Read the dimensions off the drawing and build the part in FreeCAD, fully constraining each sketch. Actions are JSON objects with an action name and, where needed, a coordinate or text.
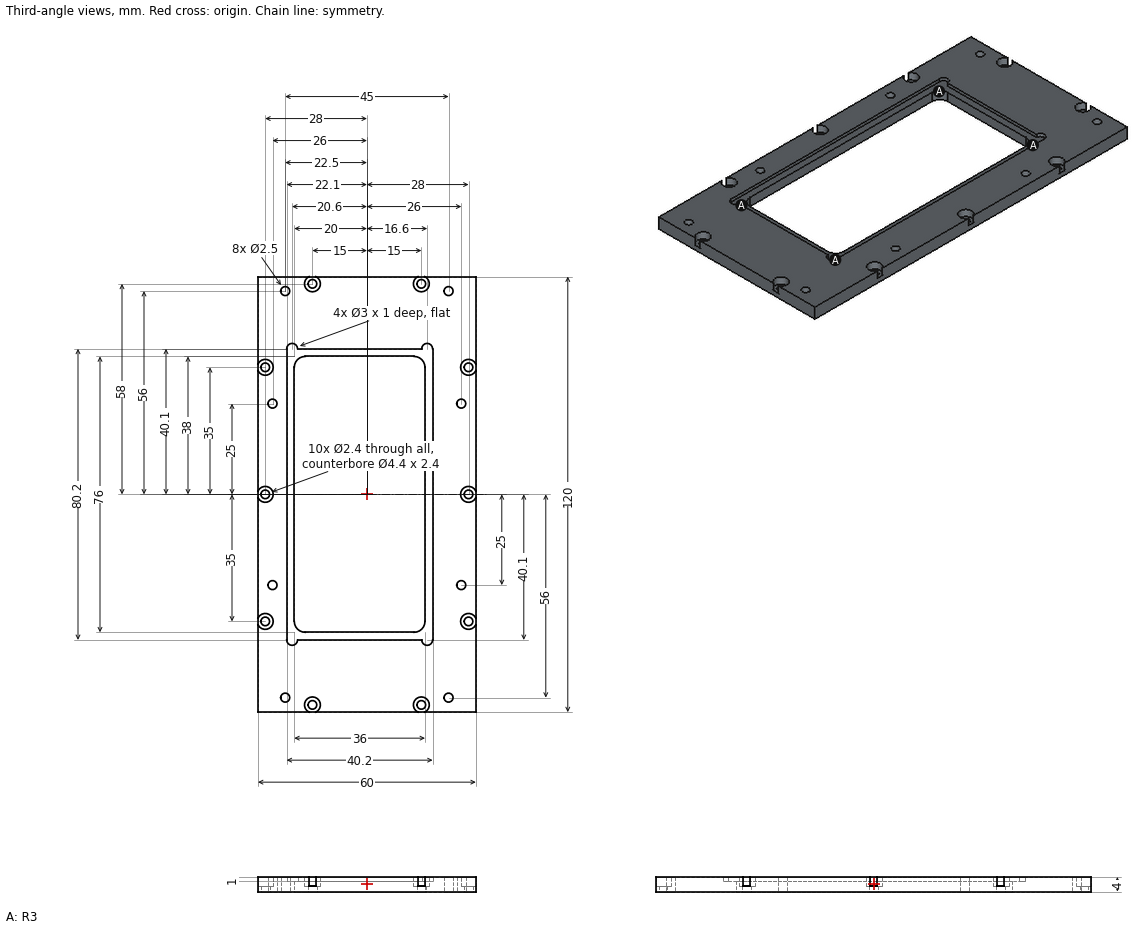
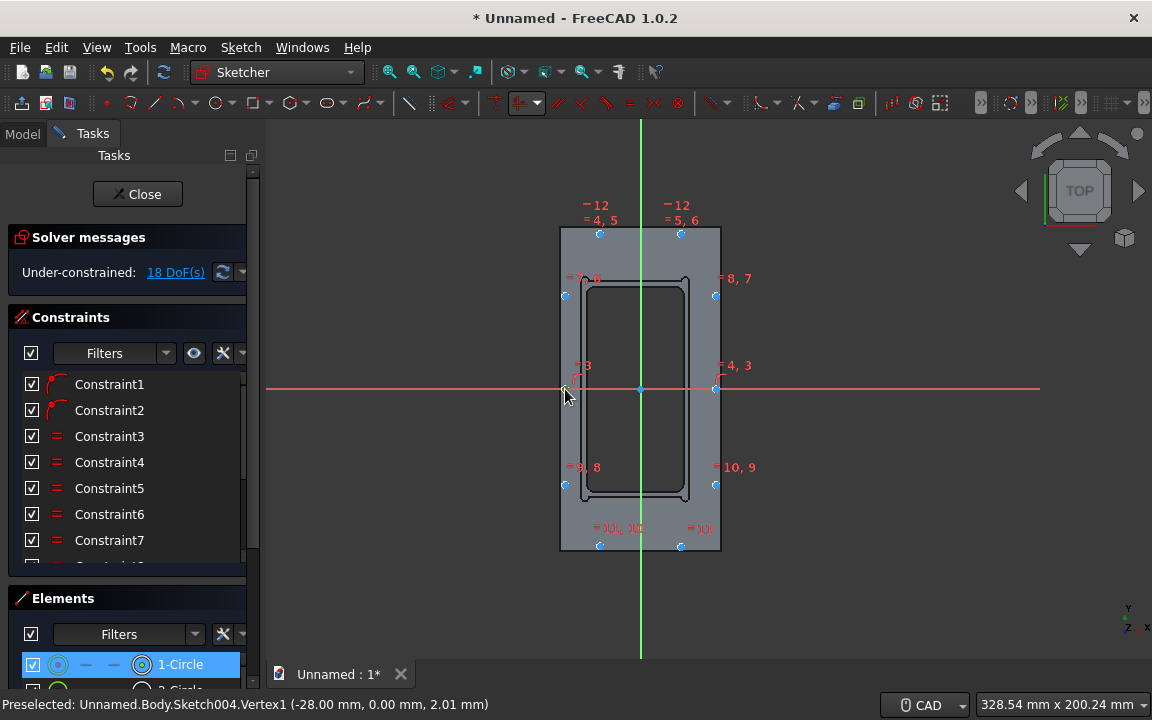
{"action": "left_click", "coordinate": [565, 296]}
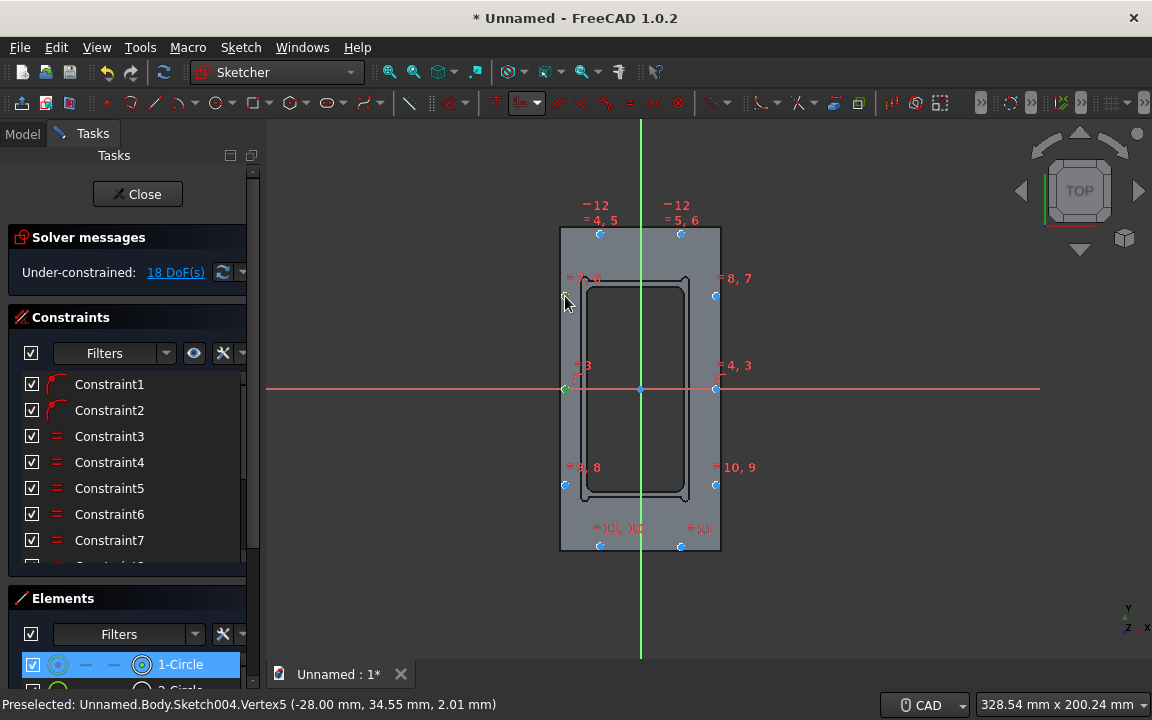
{"action": "key", "text": "v"}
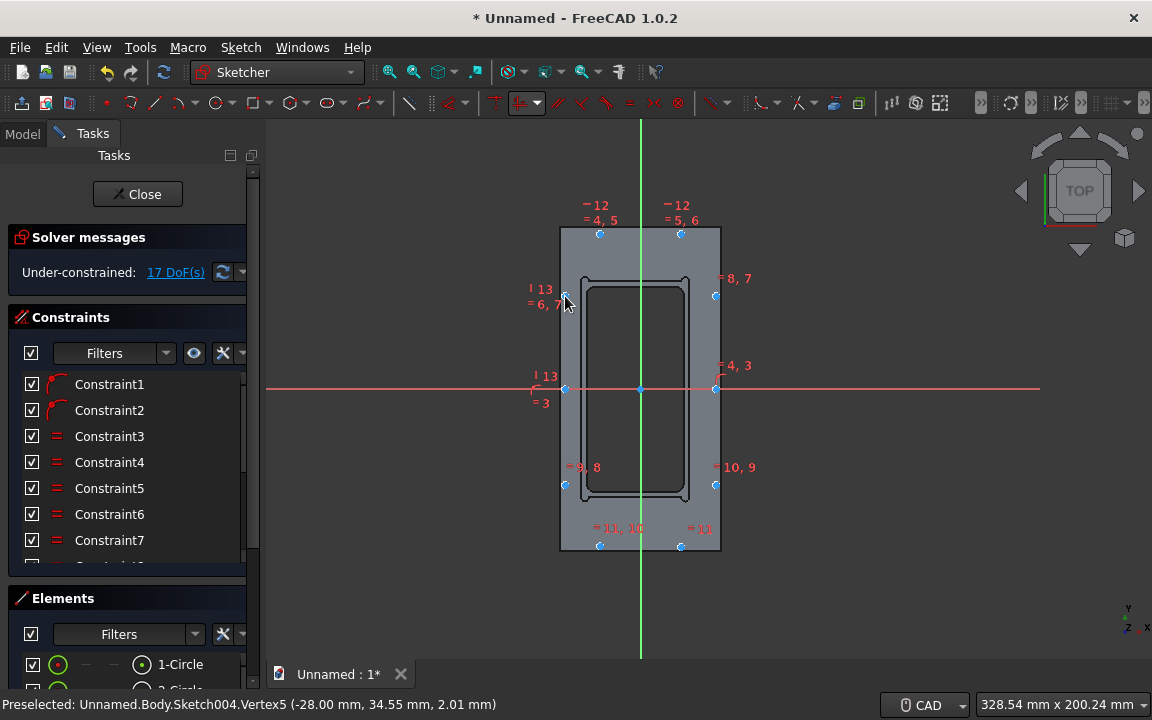
{"action": "left_click", "coordinate": [716, 389]}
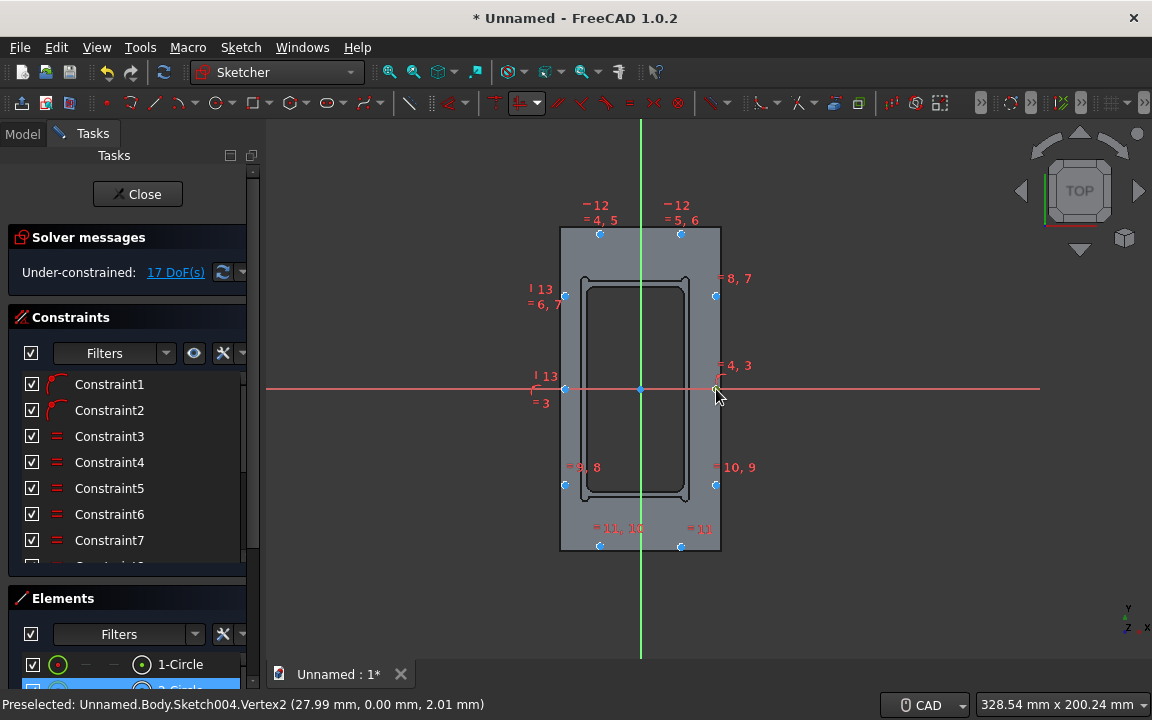
{"action": "left_click", "coordinate": [716, 296]}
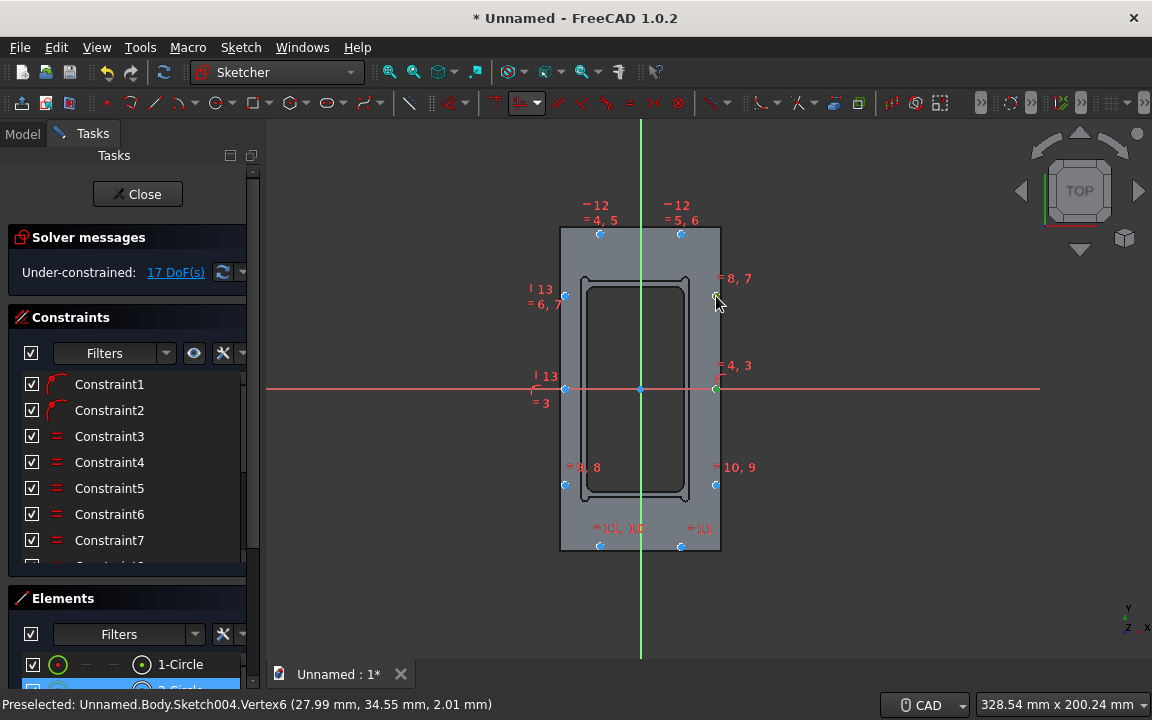
{"action": "left_click", "coordinate": [540, 104]}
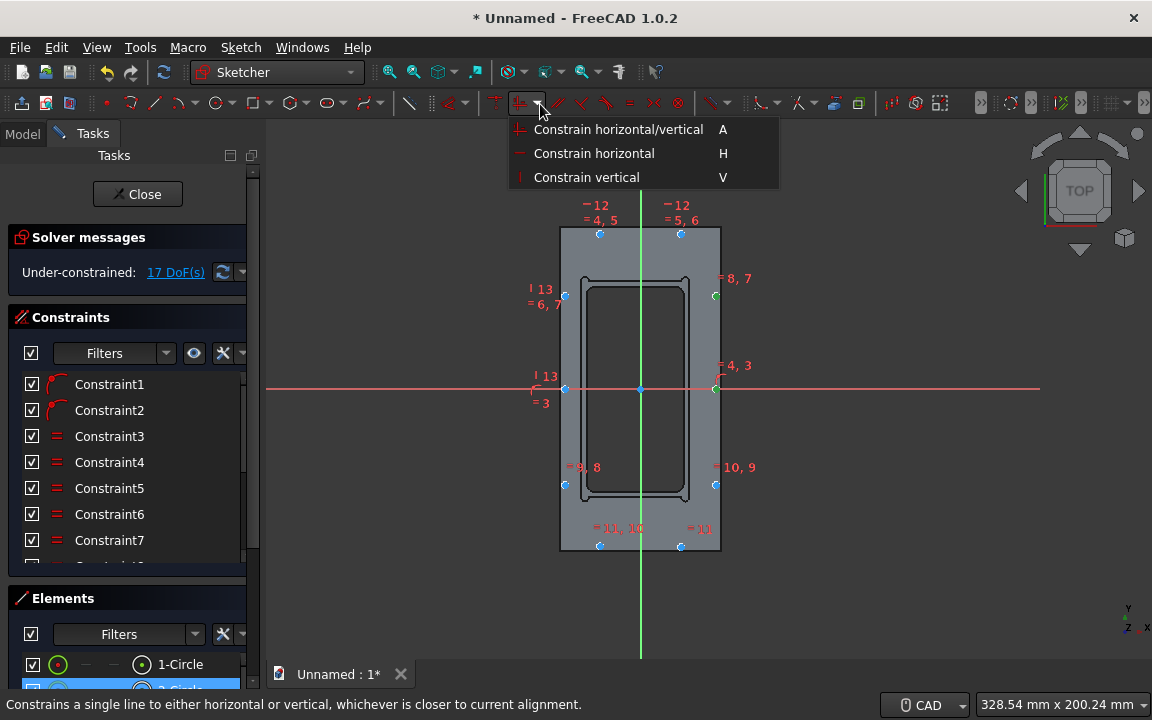
{"action": "left_click", "coordinate": [644, 177]}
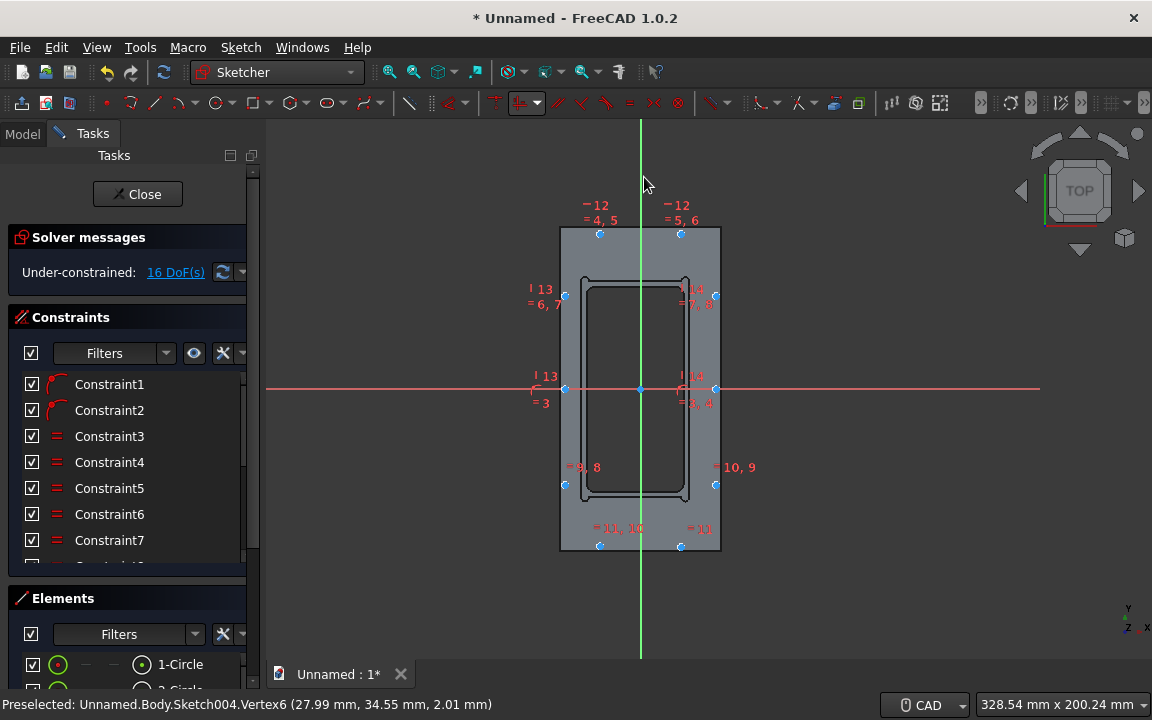
{"action": "left_click", "coordinate": [565, 296]}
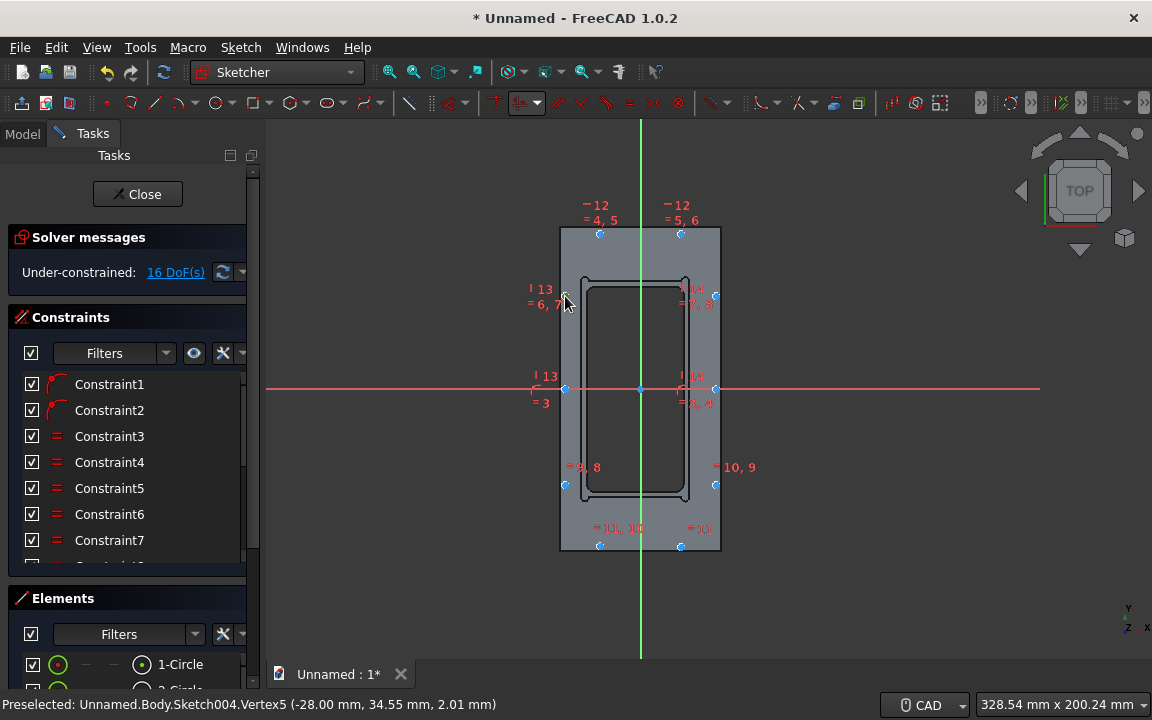
{"action": "left_click", "coordinate": [716, 296]}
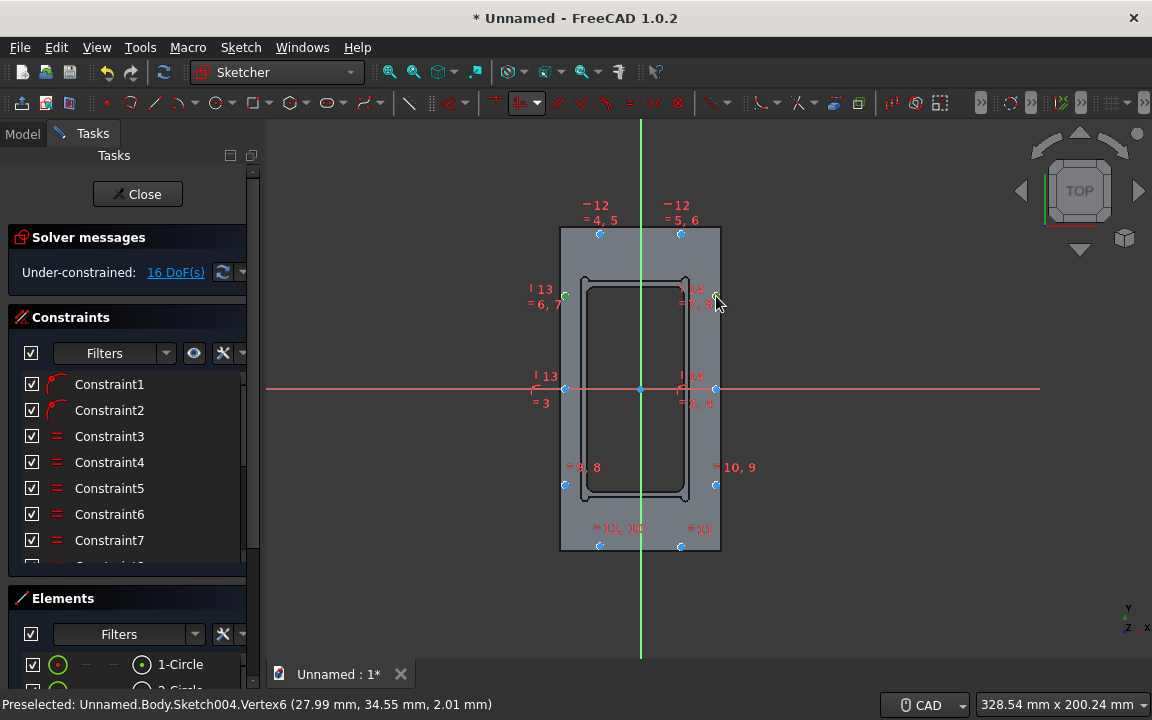
{"action": "key", "text": "h"}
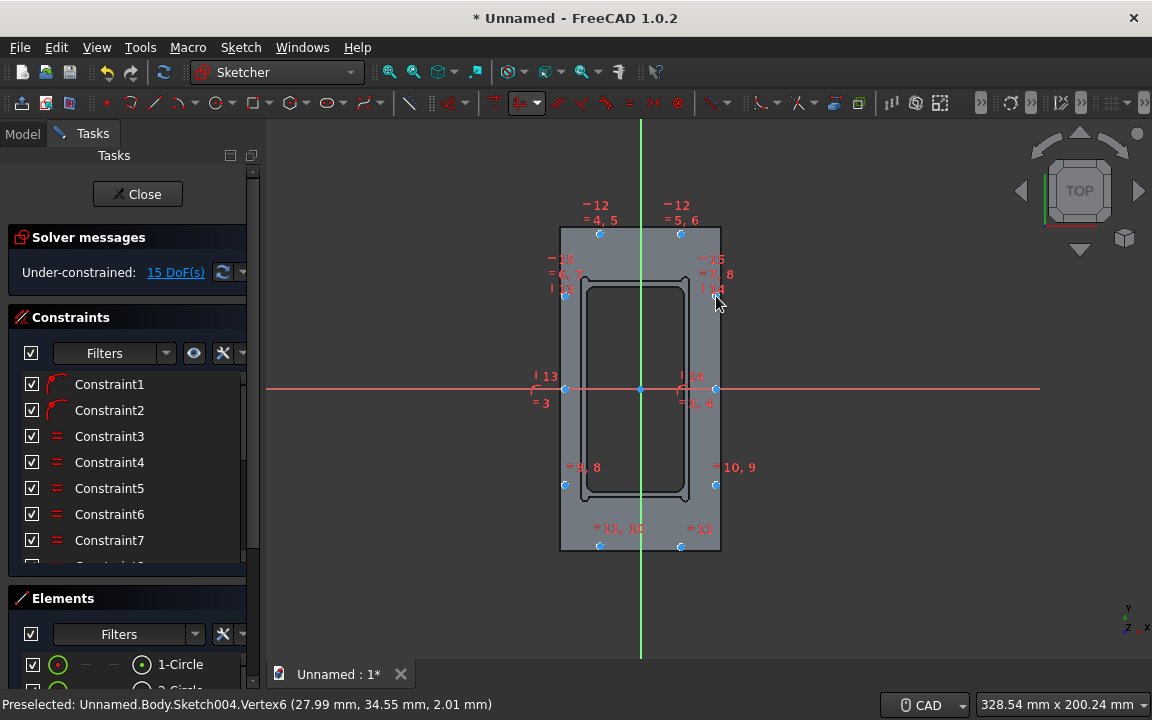
{"action": "left_click", "coordinate": [565, 389]}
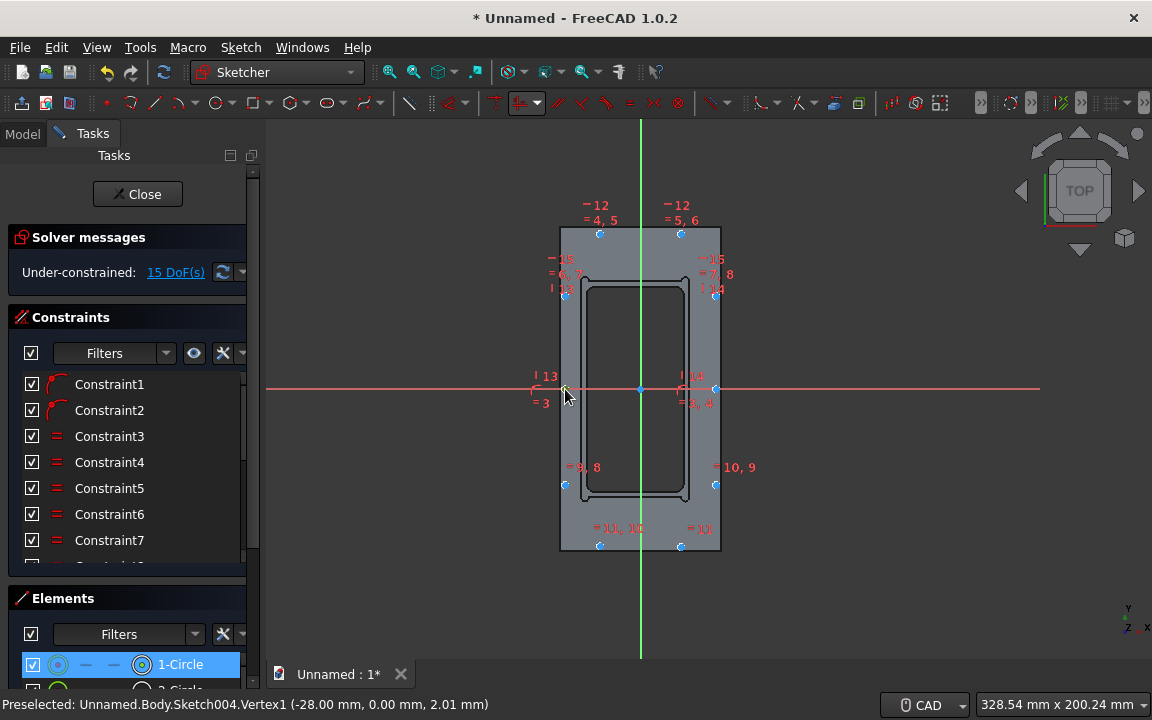
{"action": "left_click", "coordinate": [565, 485]}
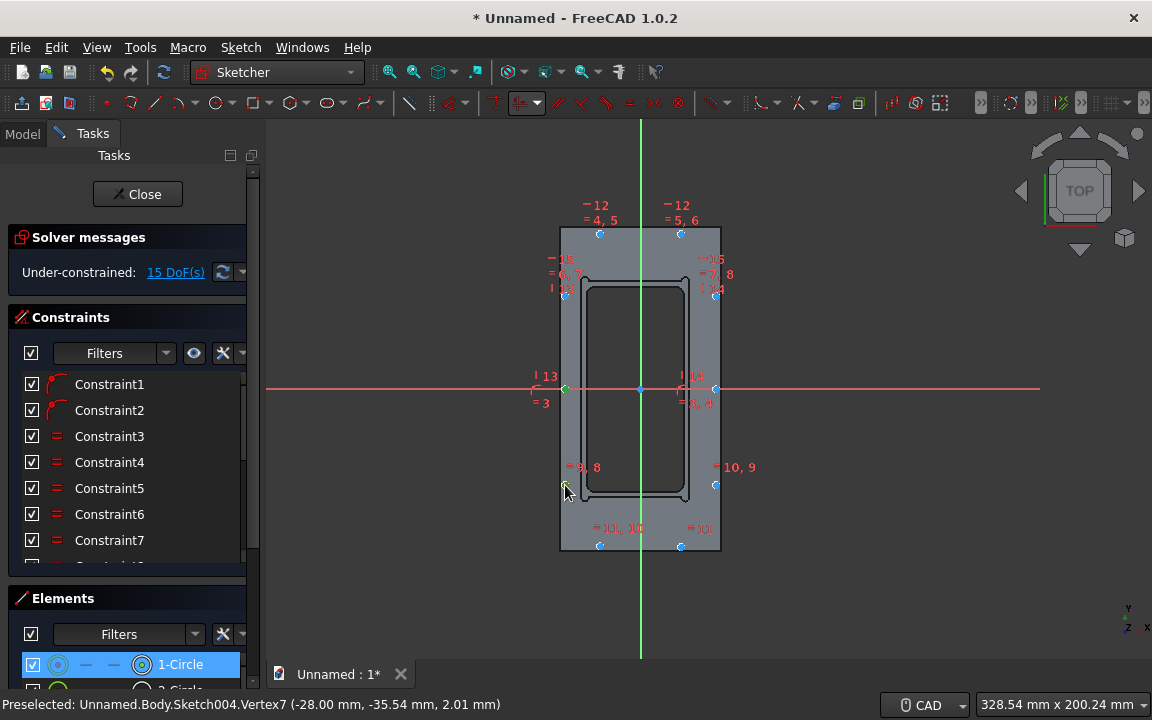
{"action": "left_click", "coordinate": [540, 104]}